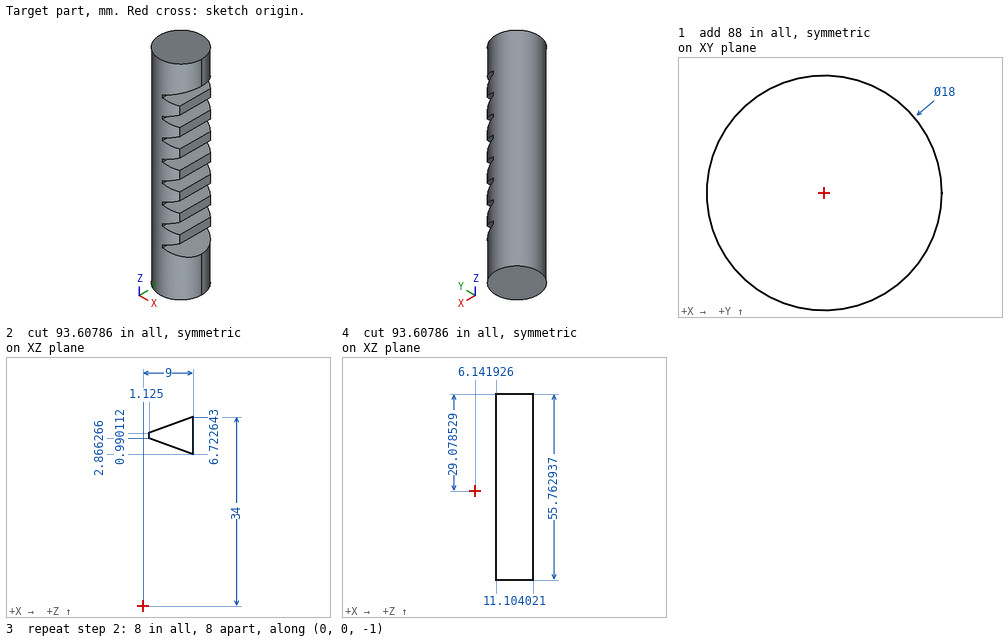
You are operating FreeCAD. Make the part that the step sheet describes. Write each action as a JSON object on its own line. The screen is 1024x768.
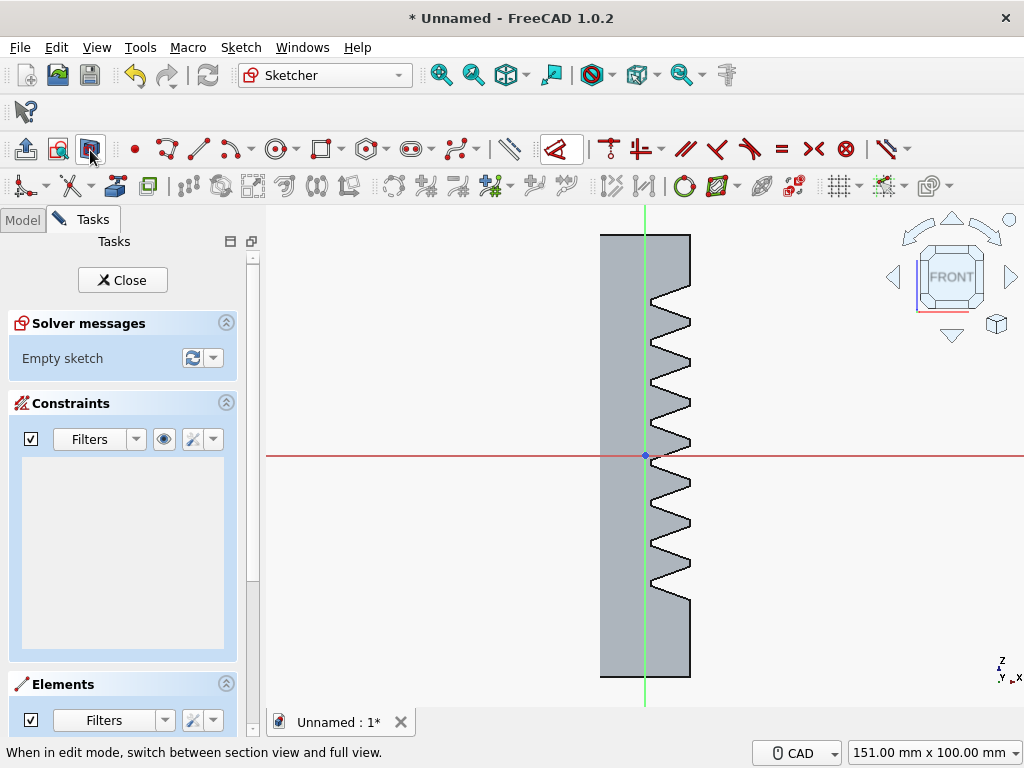
{"action": "left_click", "coordinate": [322, 150]}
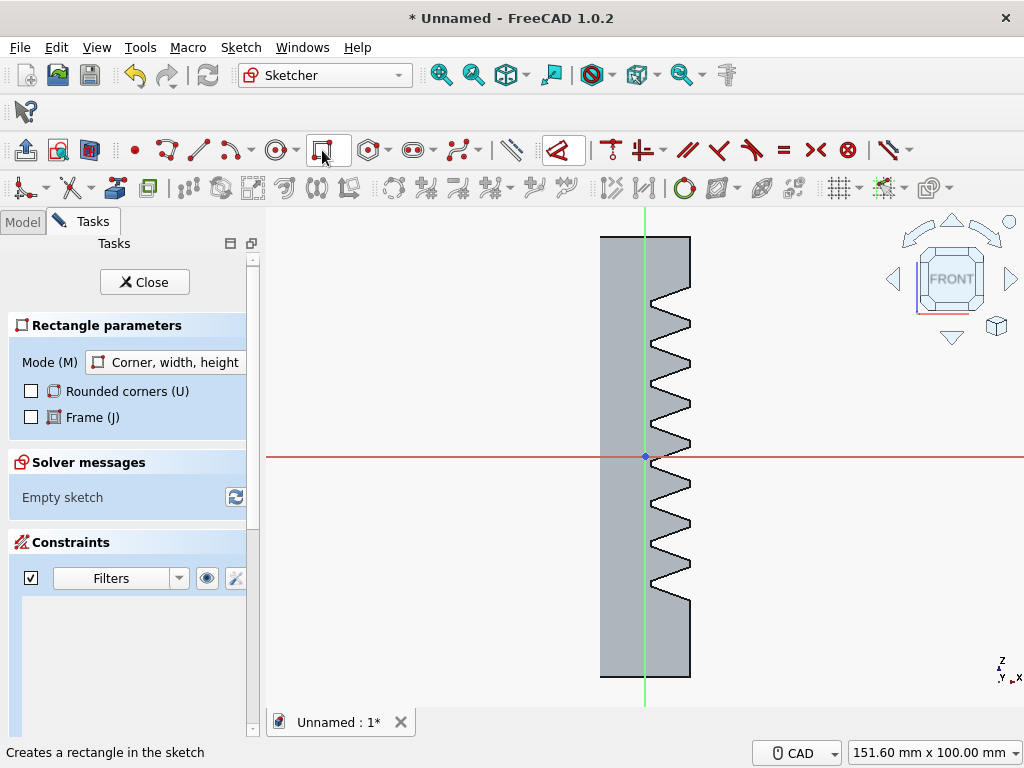
{"action": "left_click", "coordinate": [676, 312]}
{"action": "mouse_move", "coordinate": [731, 590]}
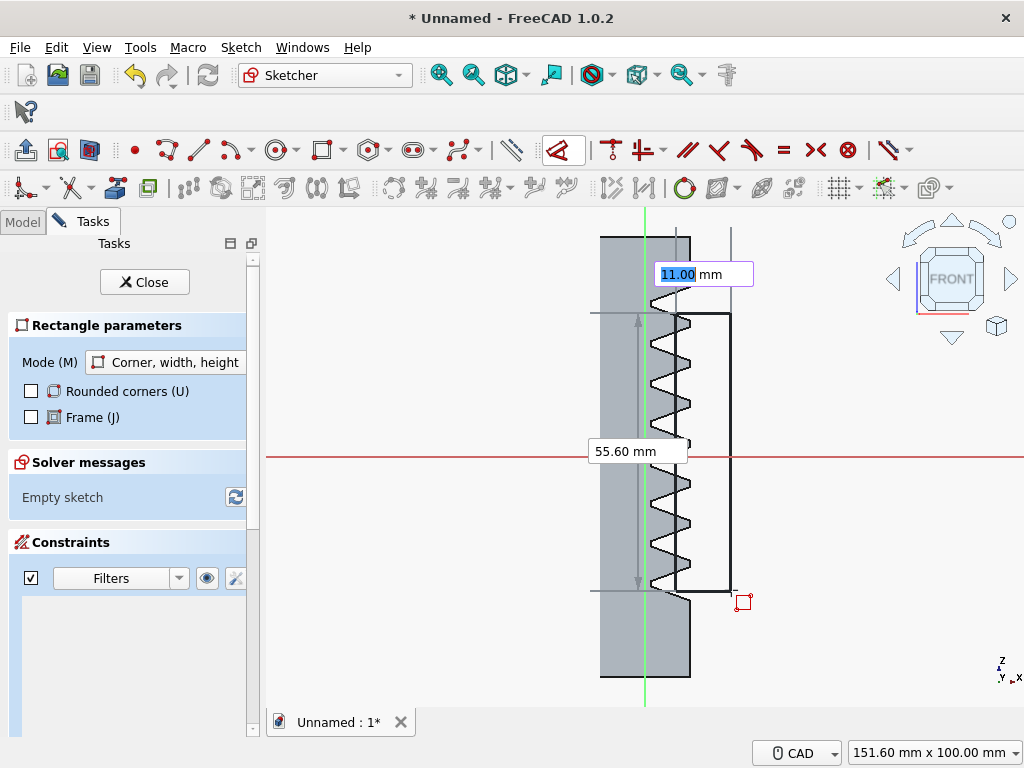
{"action": "type", "text": "11.104021"}
{"action": "key", "text": "Tab"}
{"action": "type", "text": "55.762937"}
{"action": "key", "text": "Return"}
{"action": "key", "text": "Escape"}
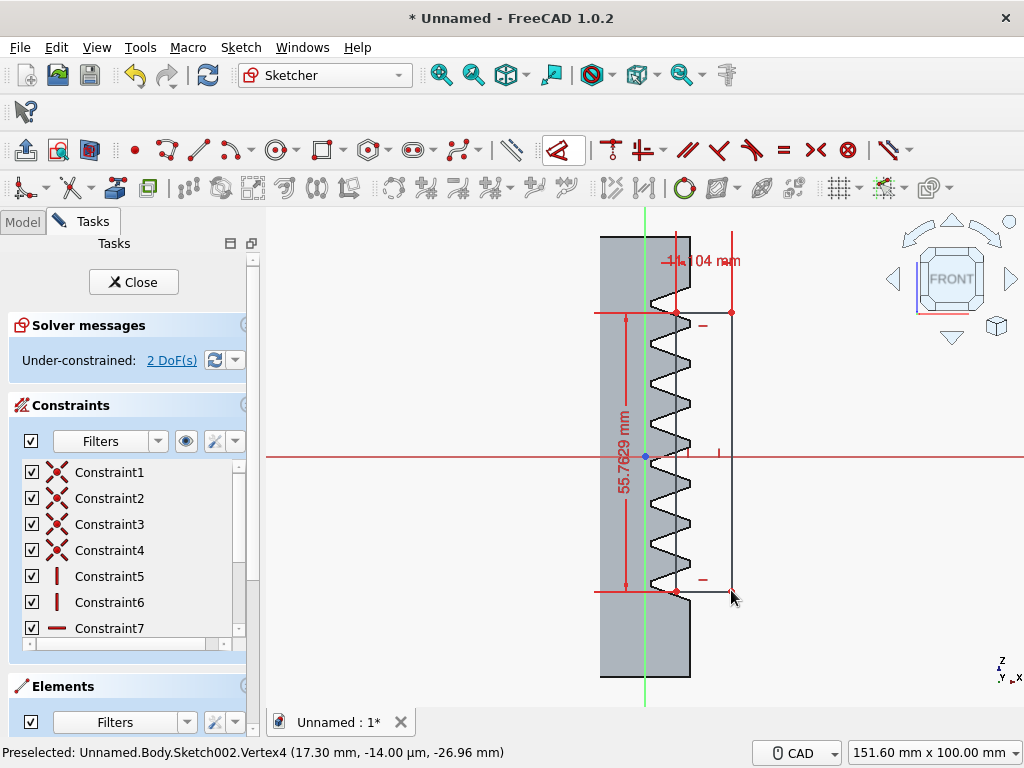
{"action": "scroll", "coordinate": [676, 313], "scroll_direction": "up", "scroll_amount": 2}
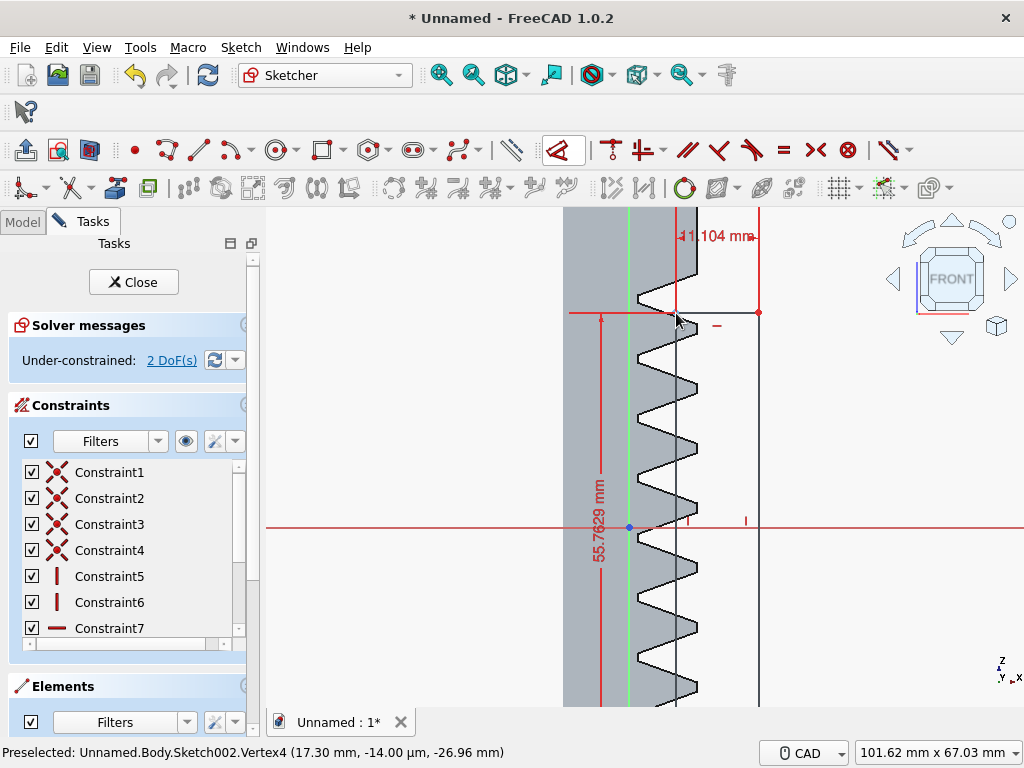
{"action": "left_click", "coordinate": [676, 313]}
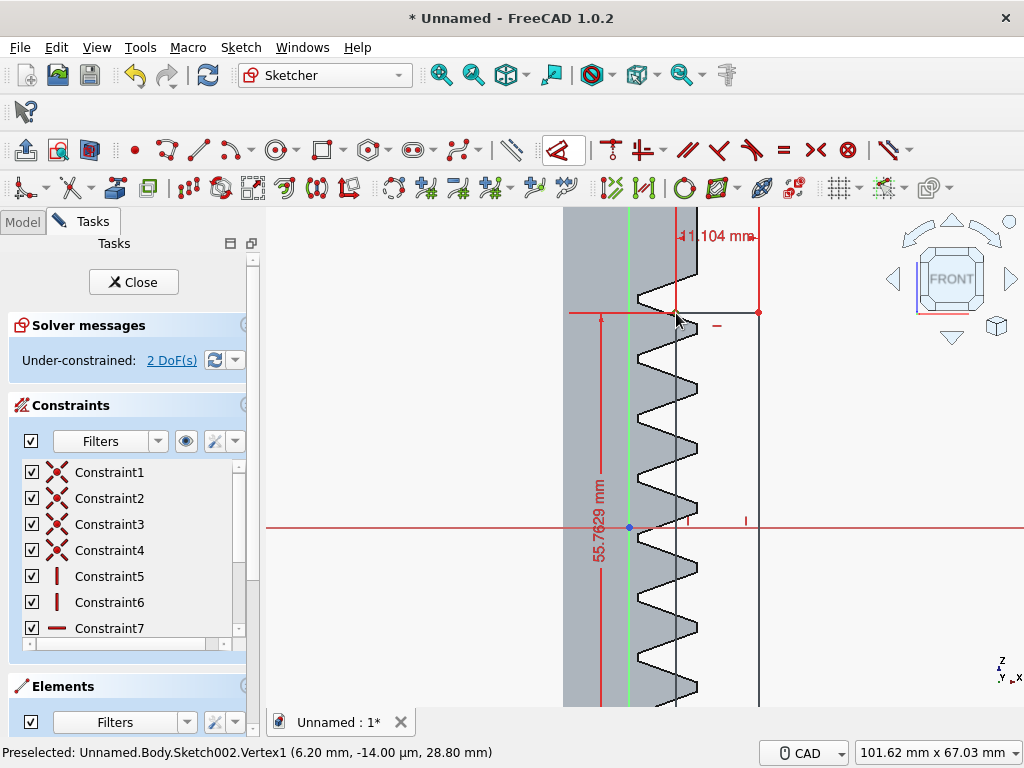
{"action": "left_click", "coordinate": [580, 150]}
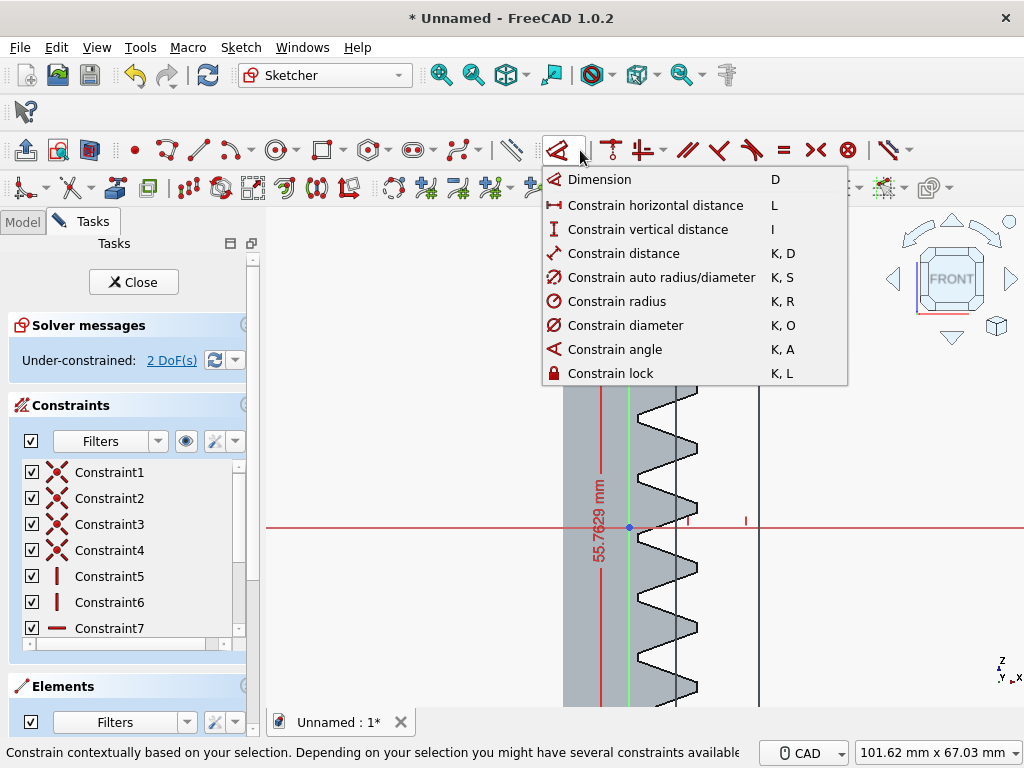
{"action": "left_click", "coordinate": [695, 205]}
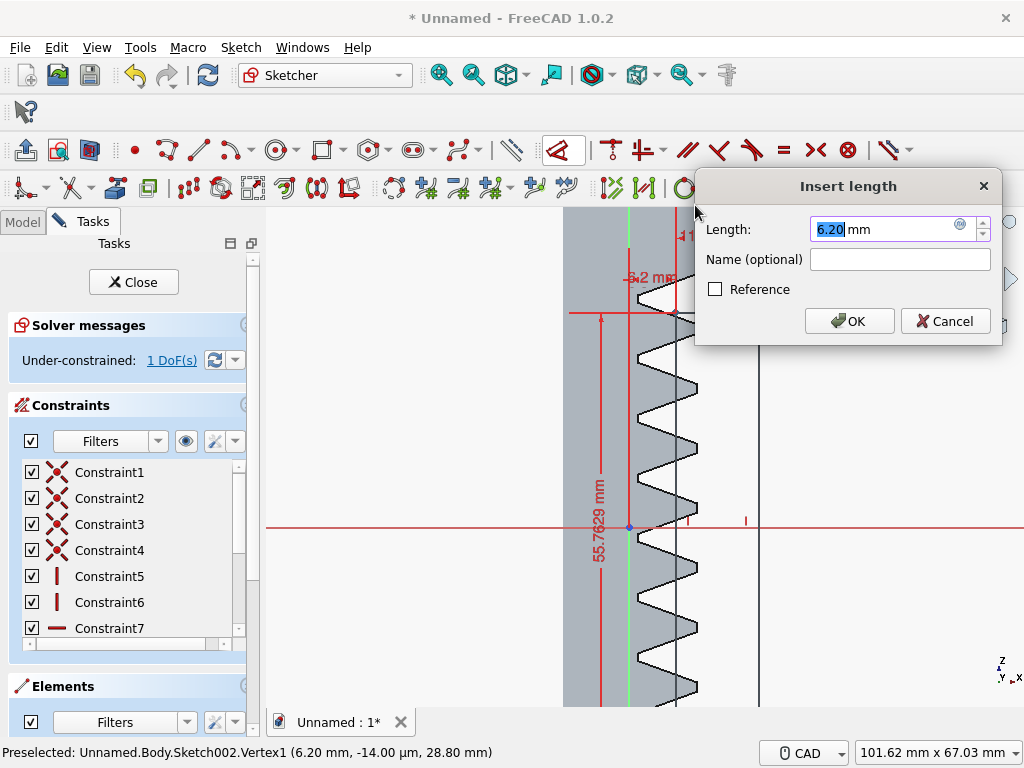
{"action": "type", "text": "6.141926"}
{"action": "key", "text": "Return"}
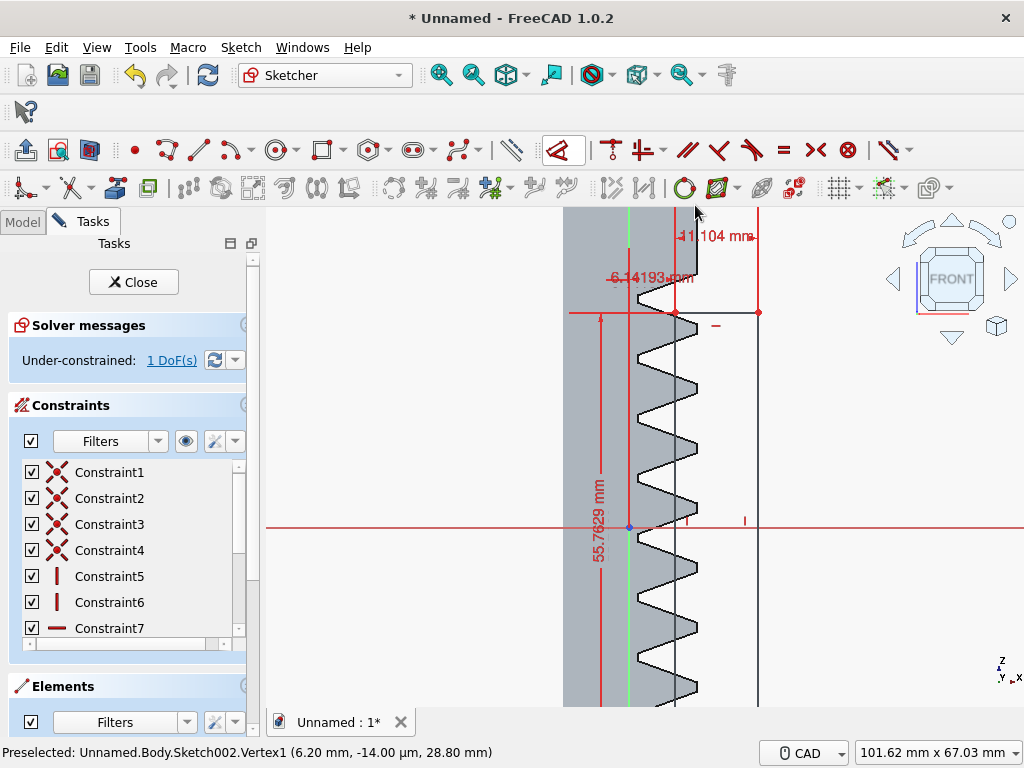
{"action": "left_click", "coordinate": [675, 313]}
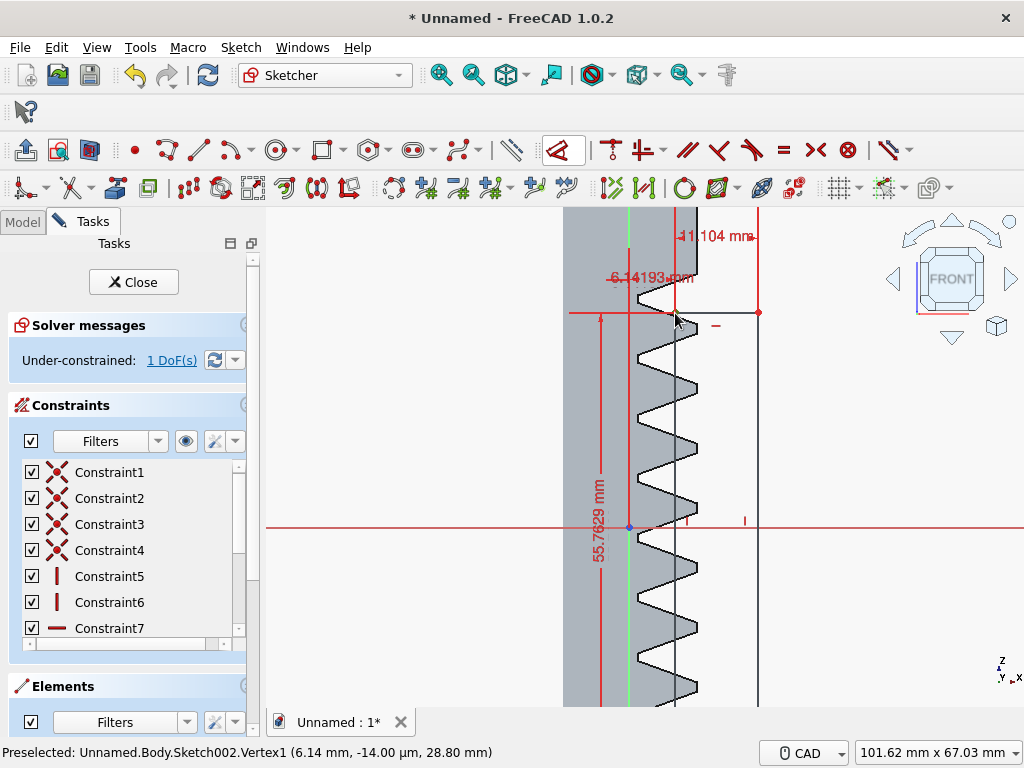
{"action": "left_click", "coordinate": [580, 150]}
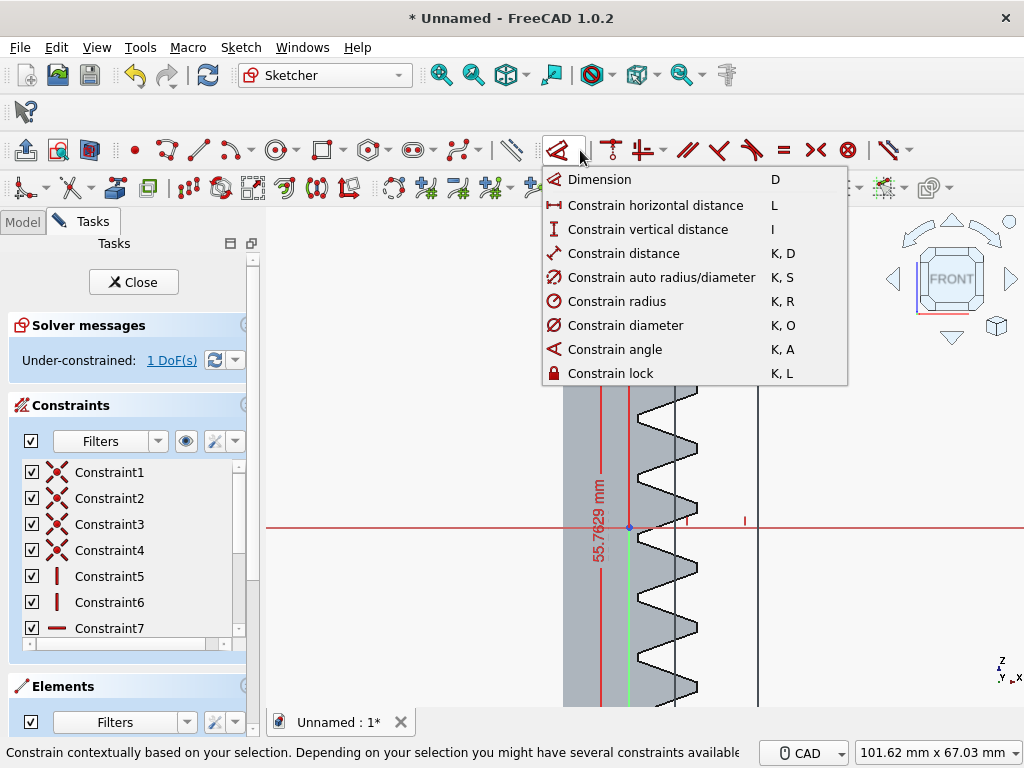
{"action": "left_click", "coordinate": [695, 229]}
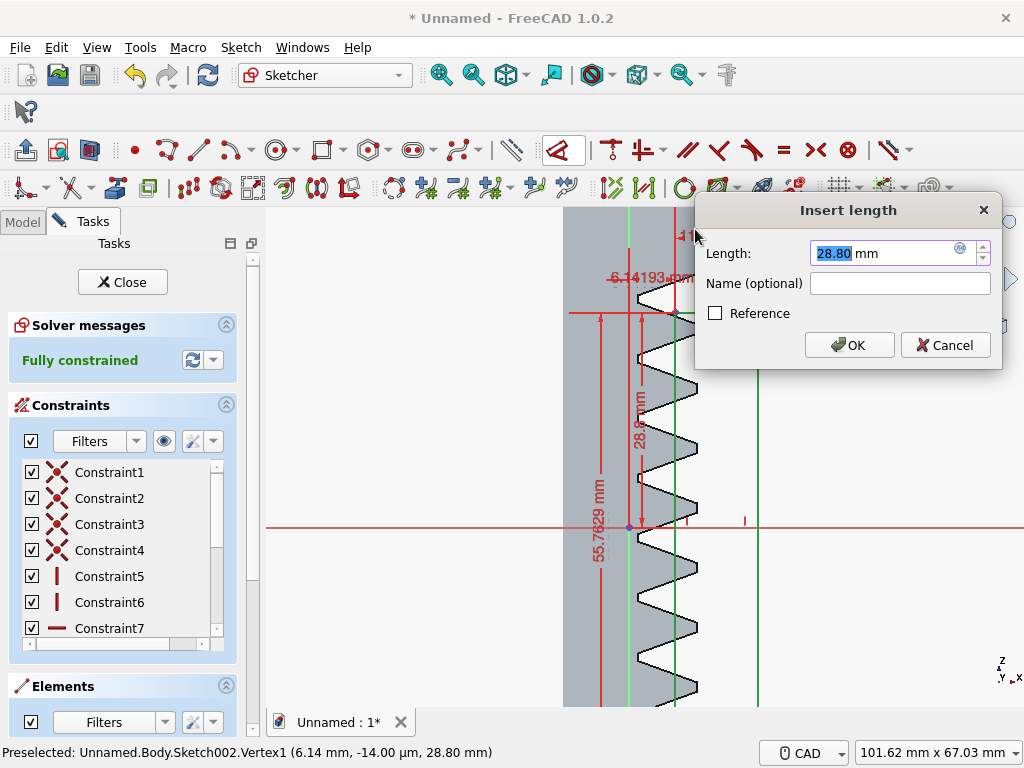
{"action": "type", "text": "29.078529"}
{"action": "key", "text": "Return"}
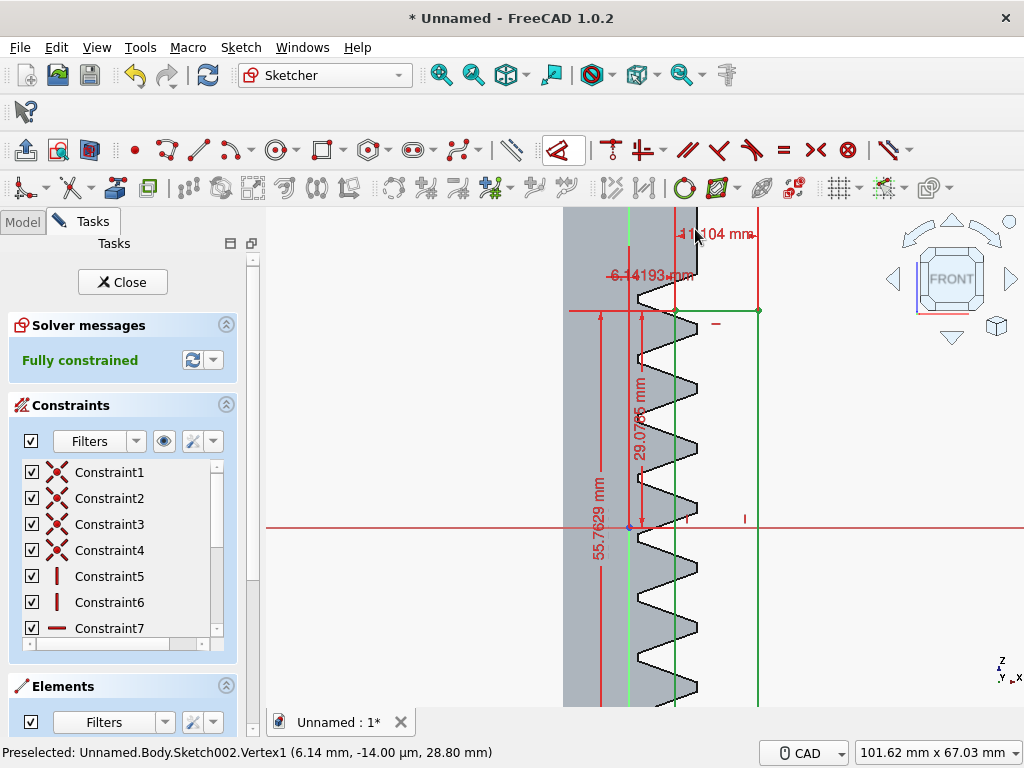
{"action": "left_click", "coordinate": [123, 282]}